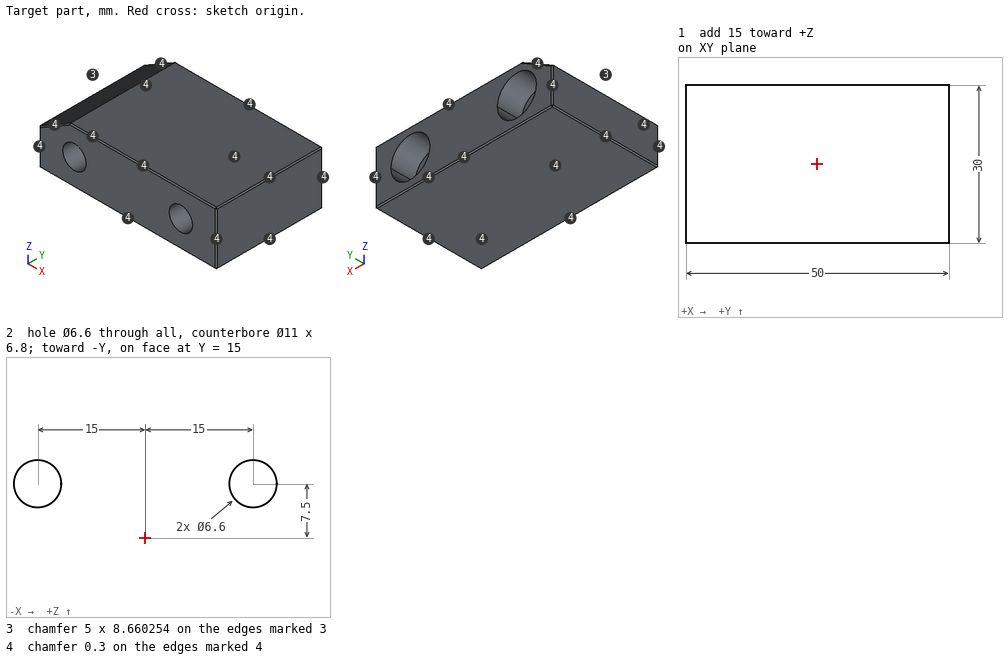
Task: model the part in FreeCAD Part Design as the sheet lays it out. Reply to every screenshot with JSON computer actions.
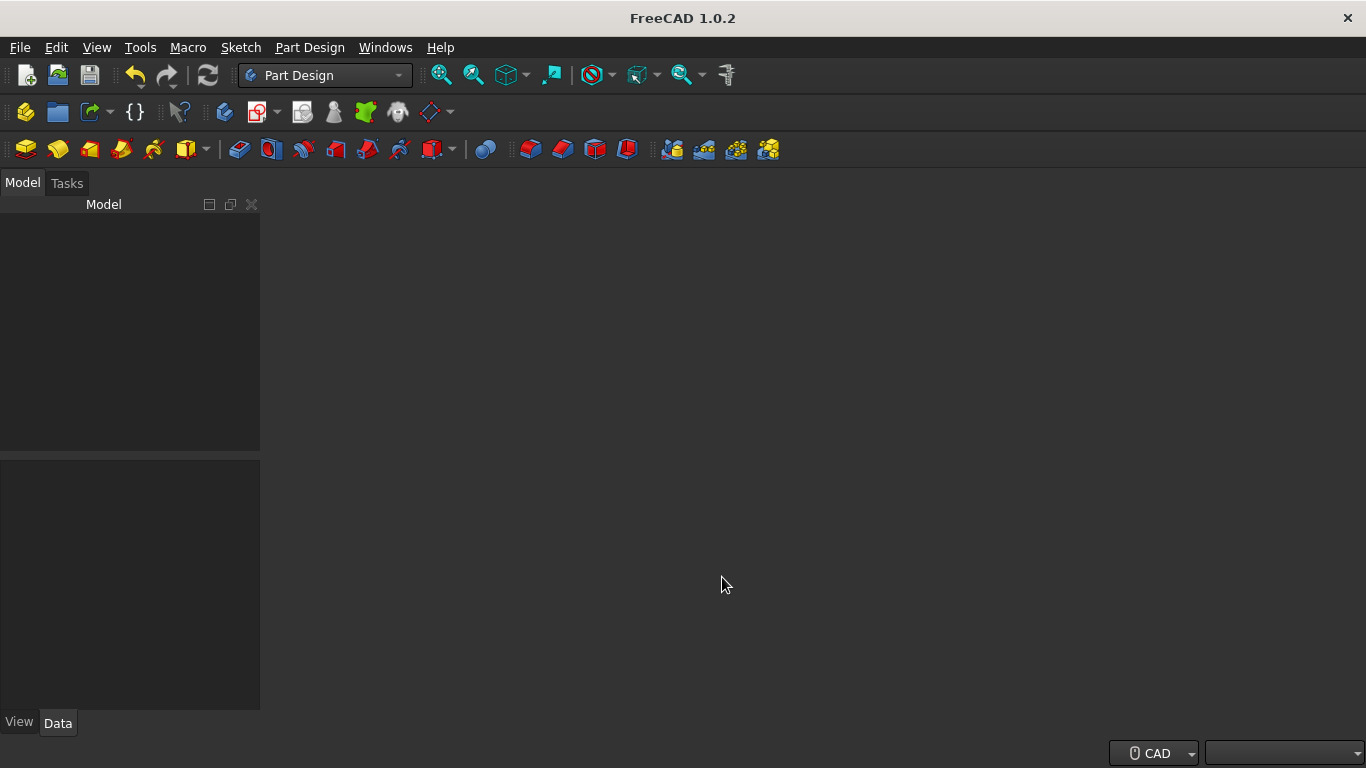
{"action": "left_click", "coordinate": [26, 76]}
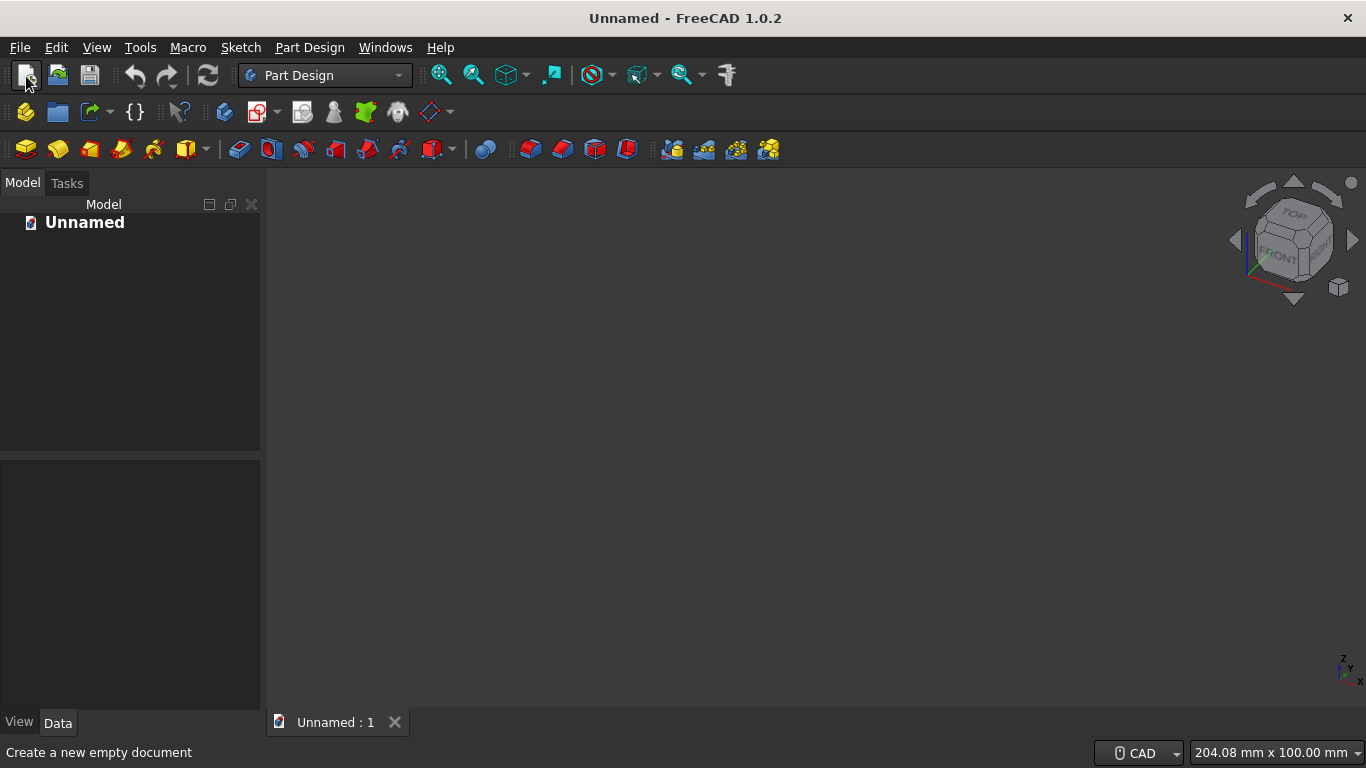
{"action": "left_click", "coordinate": [258, 112]}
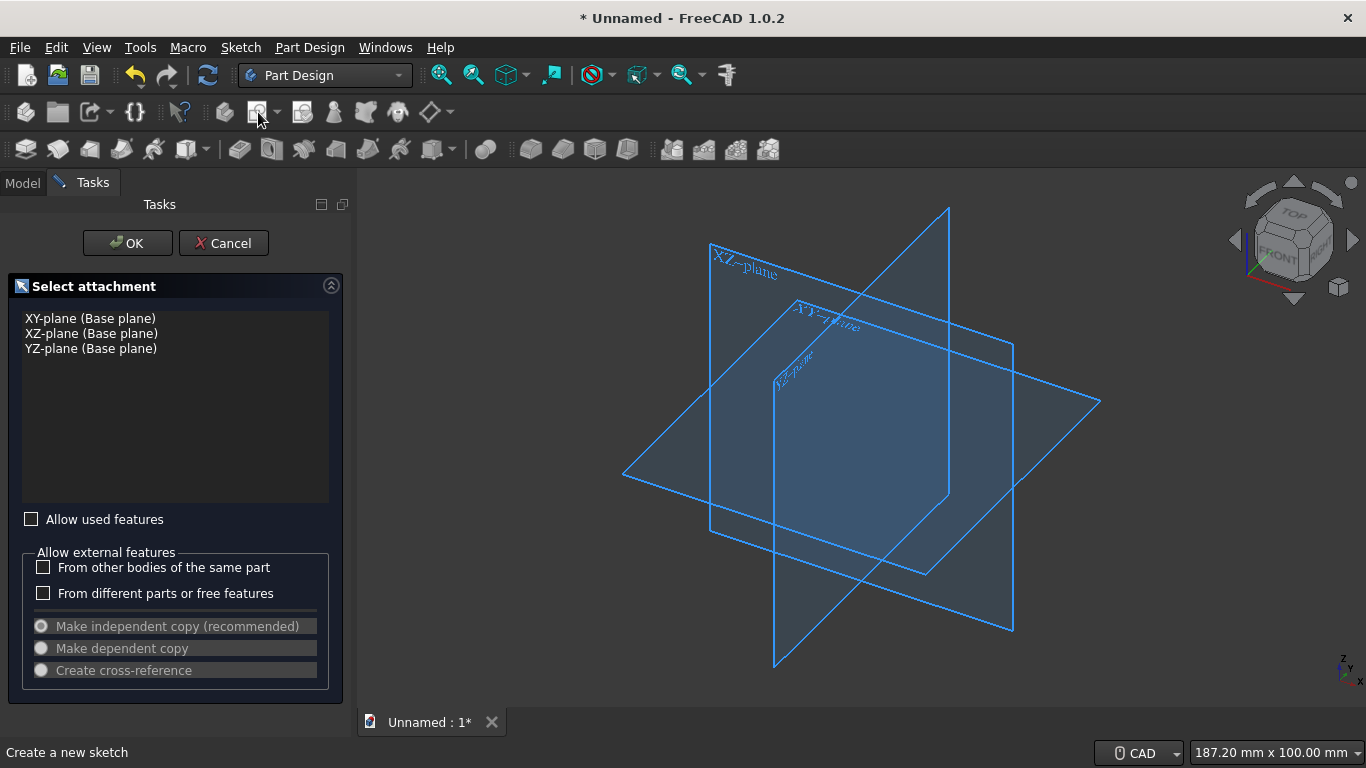
{"action": "left_click", "coordinate": [82, 318]}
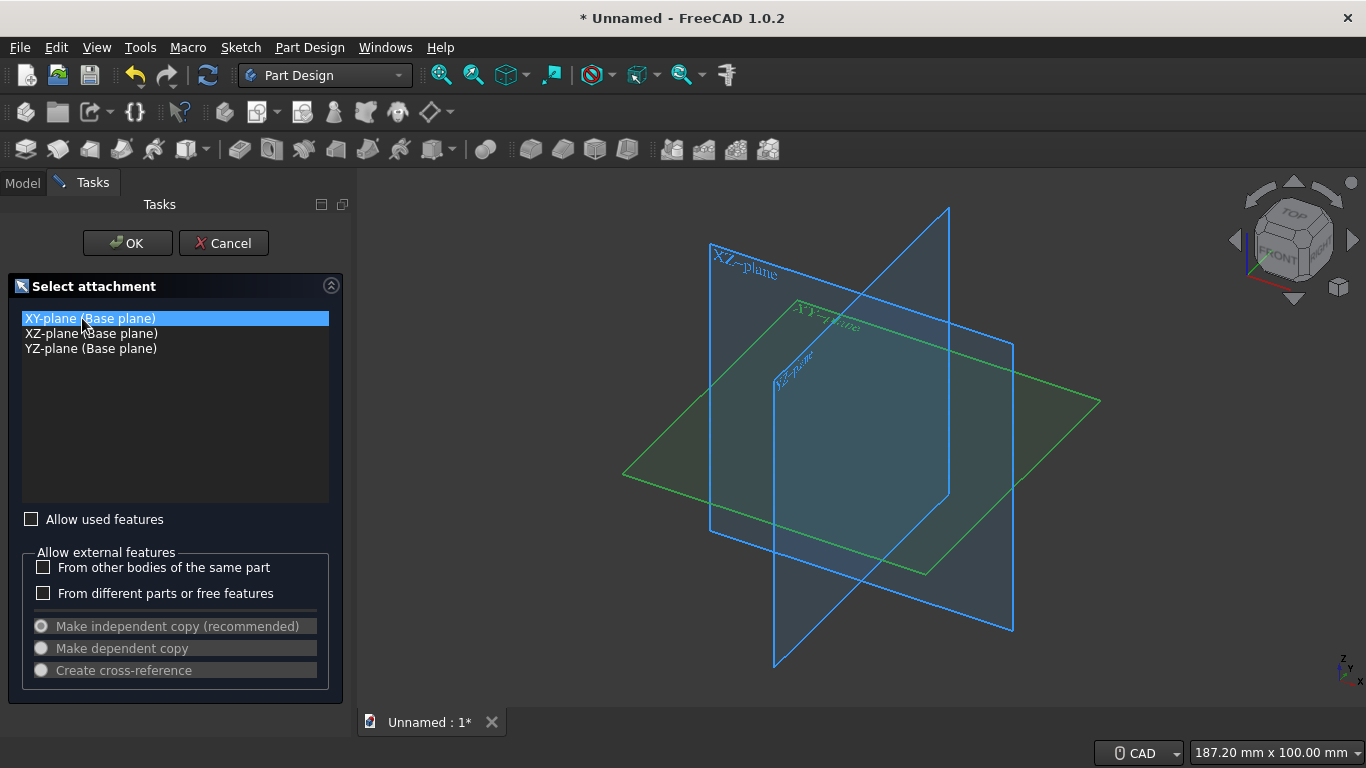
{"action": "left_click", "coordinate": [128, 243]}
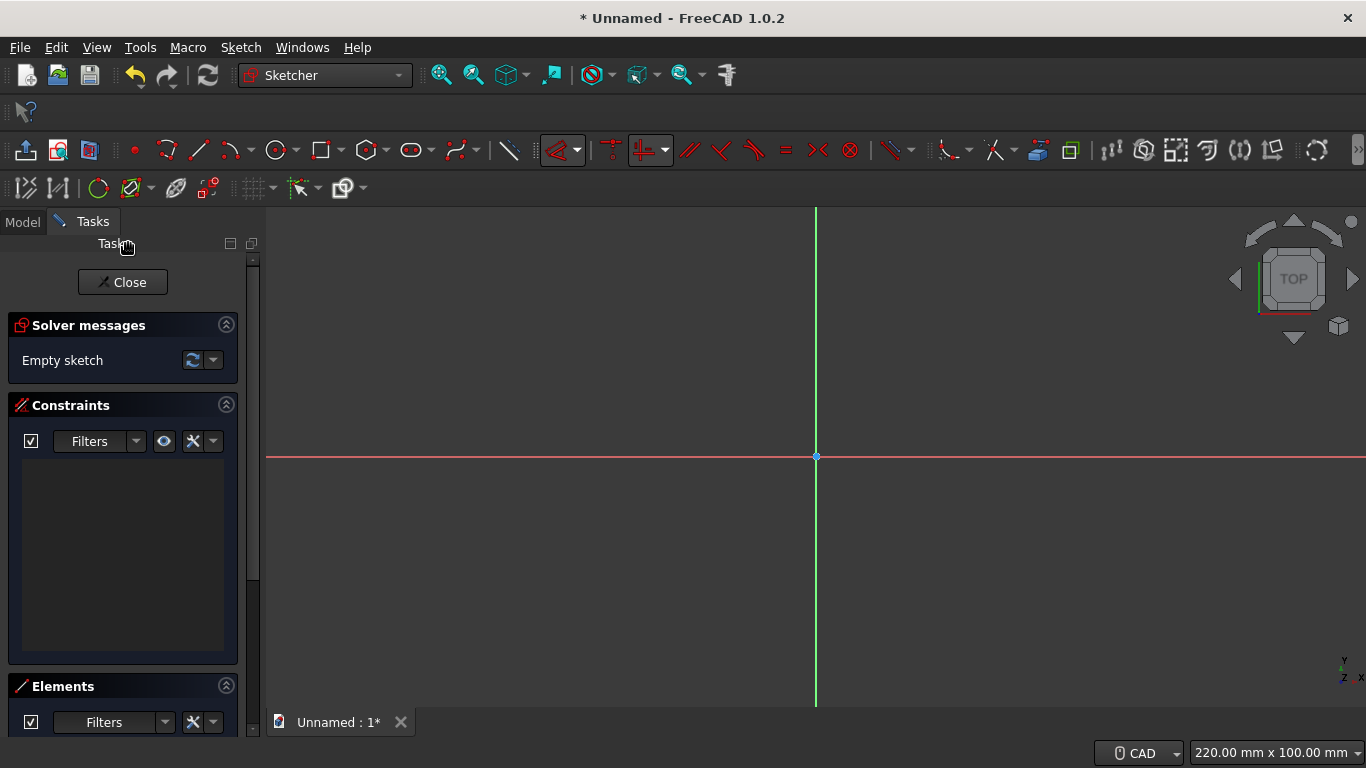
{"action": "scroll", "coordinate": [872, 457], "scroll_direction": "up", "scroll_amount": 4}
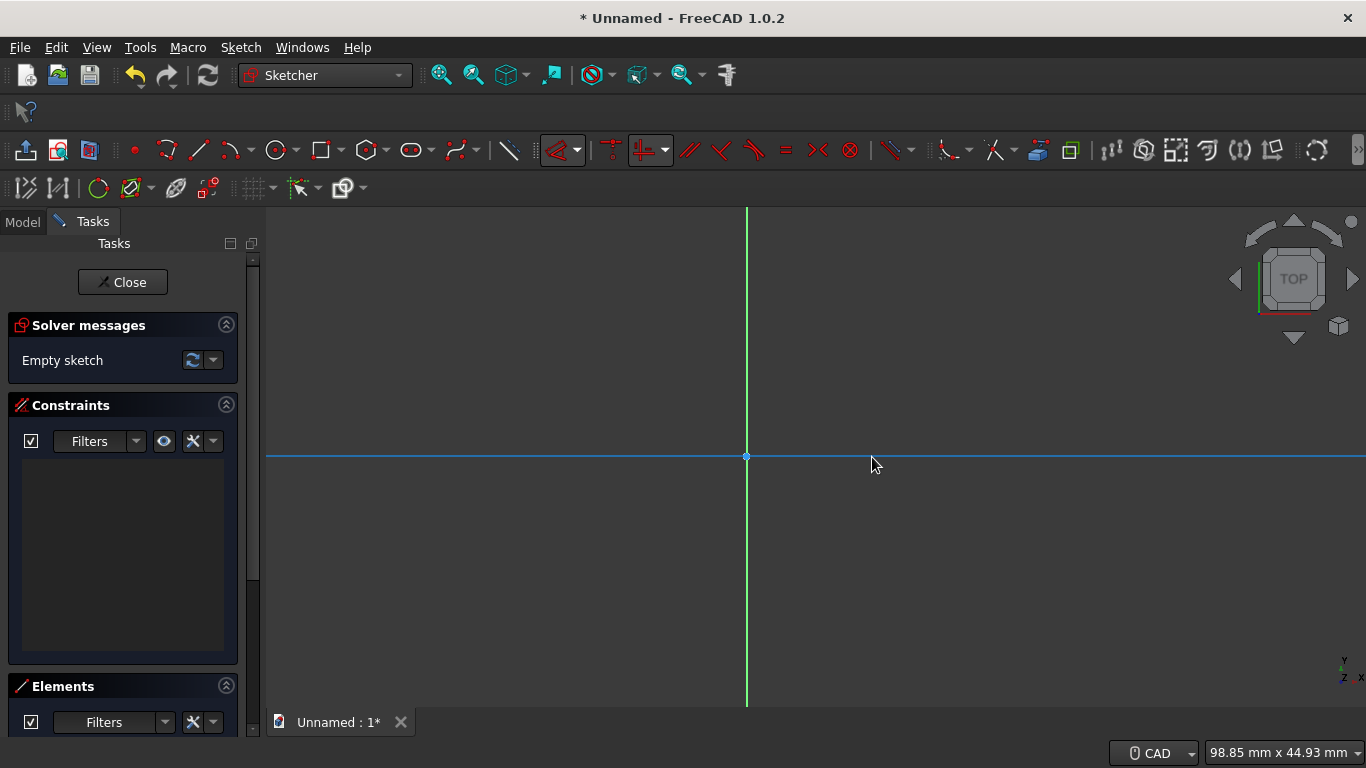
{"action": "left_click", "coordinate": [344, 150]}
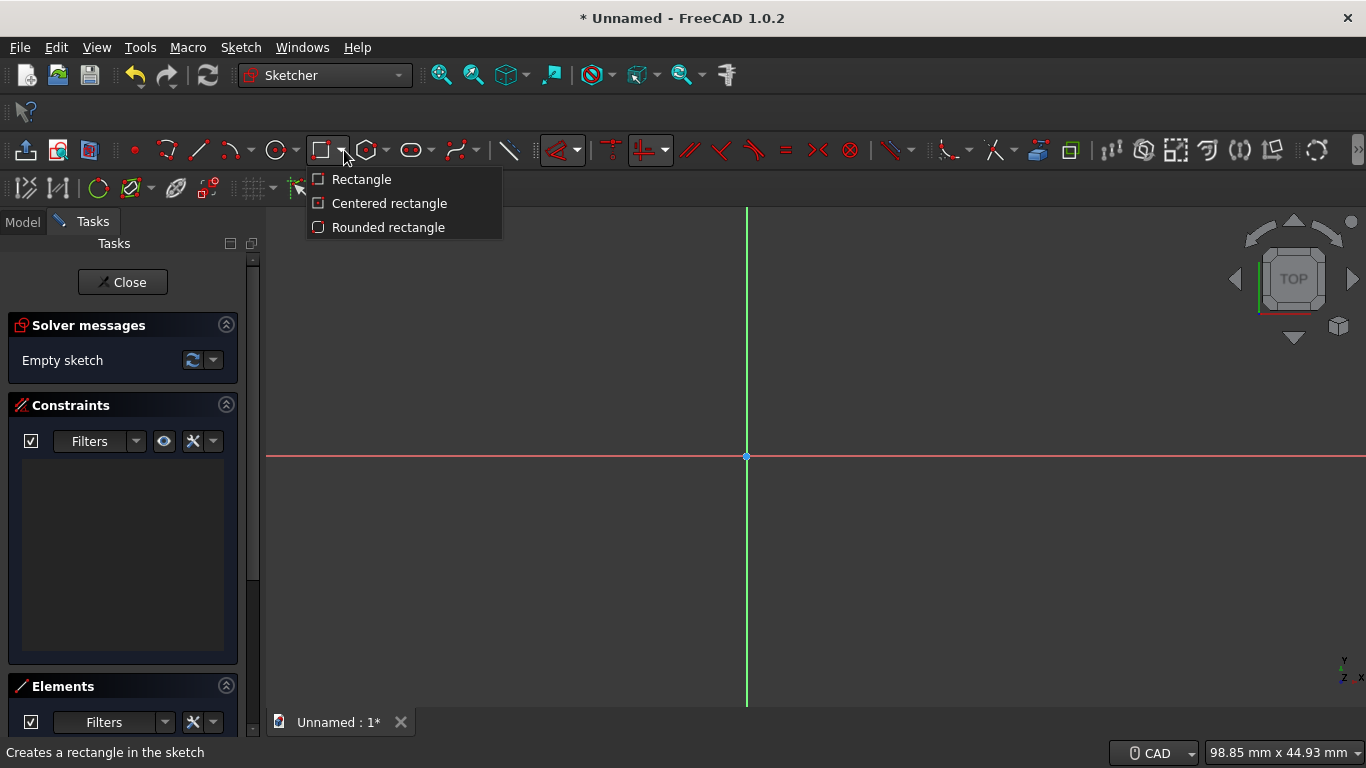
{"action": "left_click", "coordinate": [404, 203]}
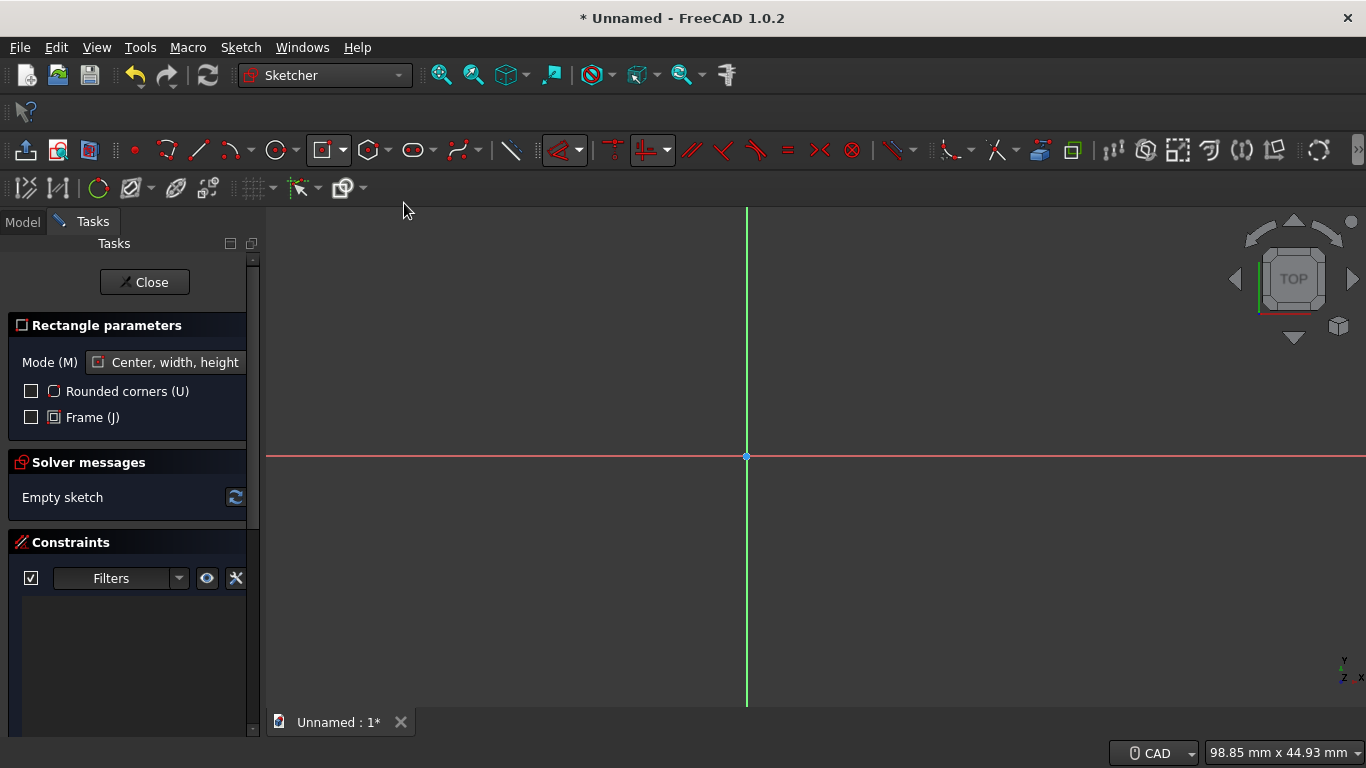
{"action": "left_click", "coordinate": [747, 456]}
{"action": "mouse_move", "coordinate": [1025, 289]}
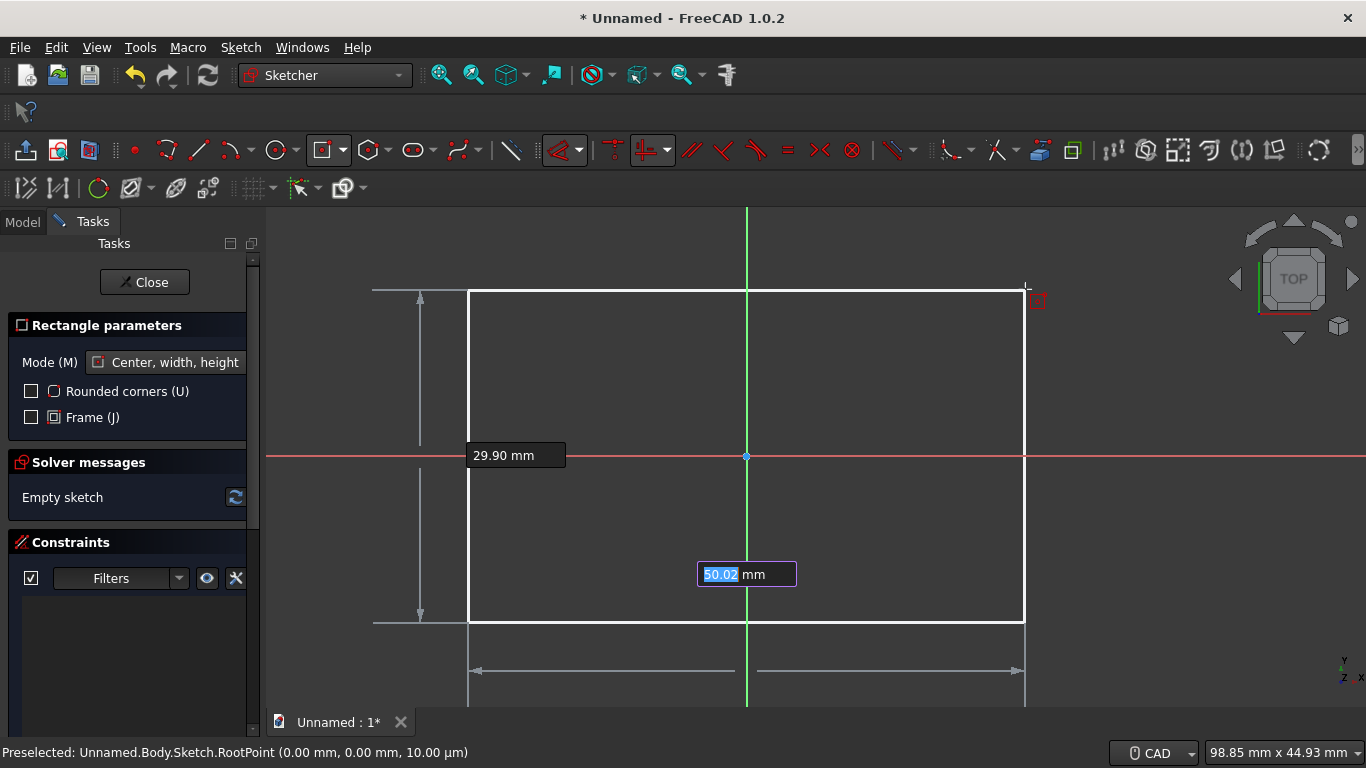
{"action": "type", "text": "50"}
{"action": "key", "text": "Tab"}
{"action": "type", "text": "30"}
{"action": "key", "text": "Return"}
{"action": "key", "text": "Escape"}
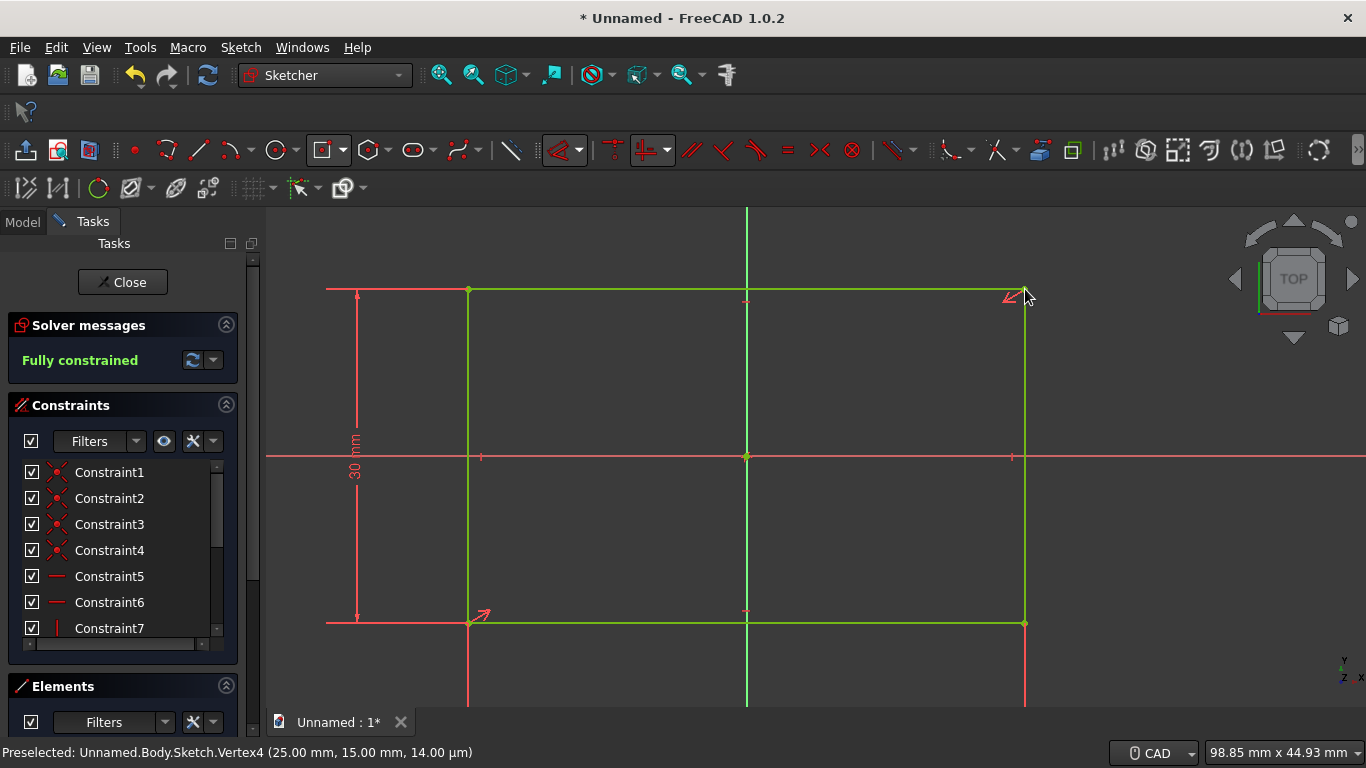
{"action": "left_click", "coordinate": [123, 282]}